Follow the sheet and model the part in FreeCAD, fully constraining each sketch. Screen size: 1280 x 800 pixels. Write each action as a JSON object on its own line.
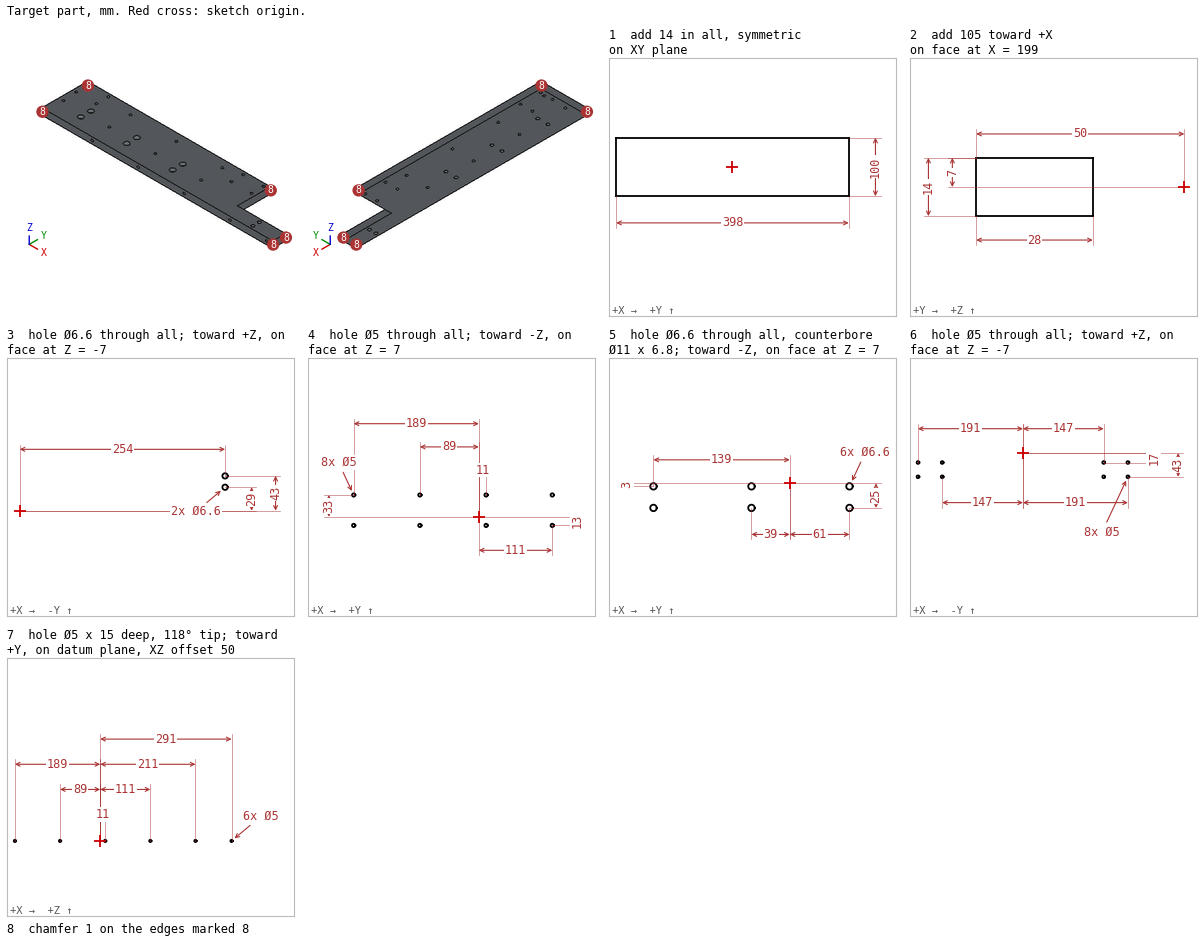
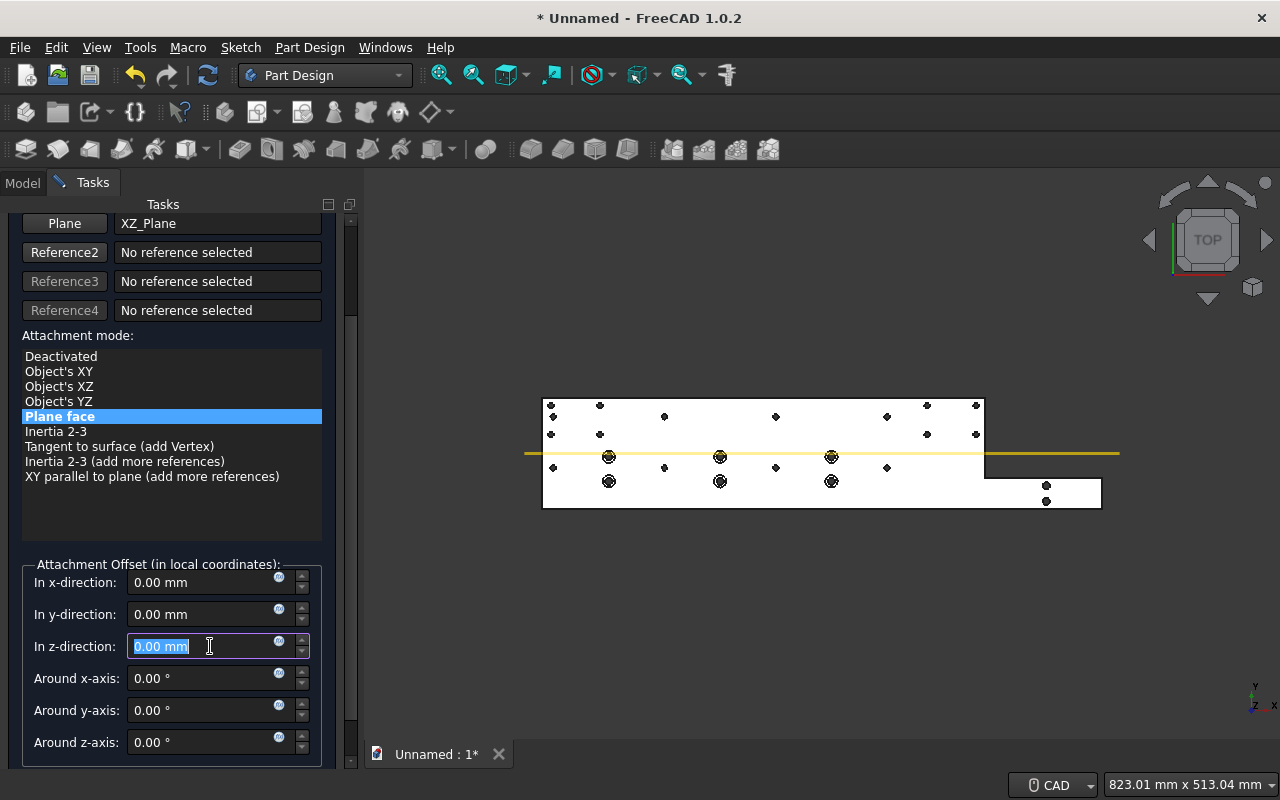
{"action": "type", "text": "50"}
{"action": "key", "text": "Tab"}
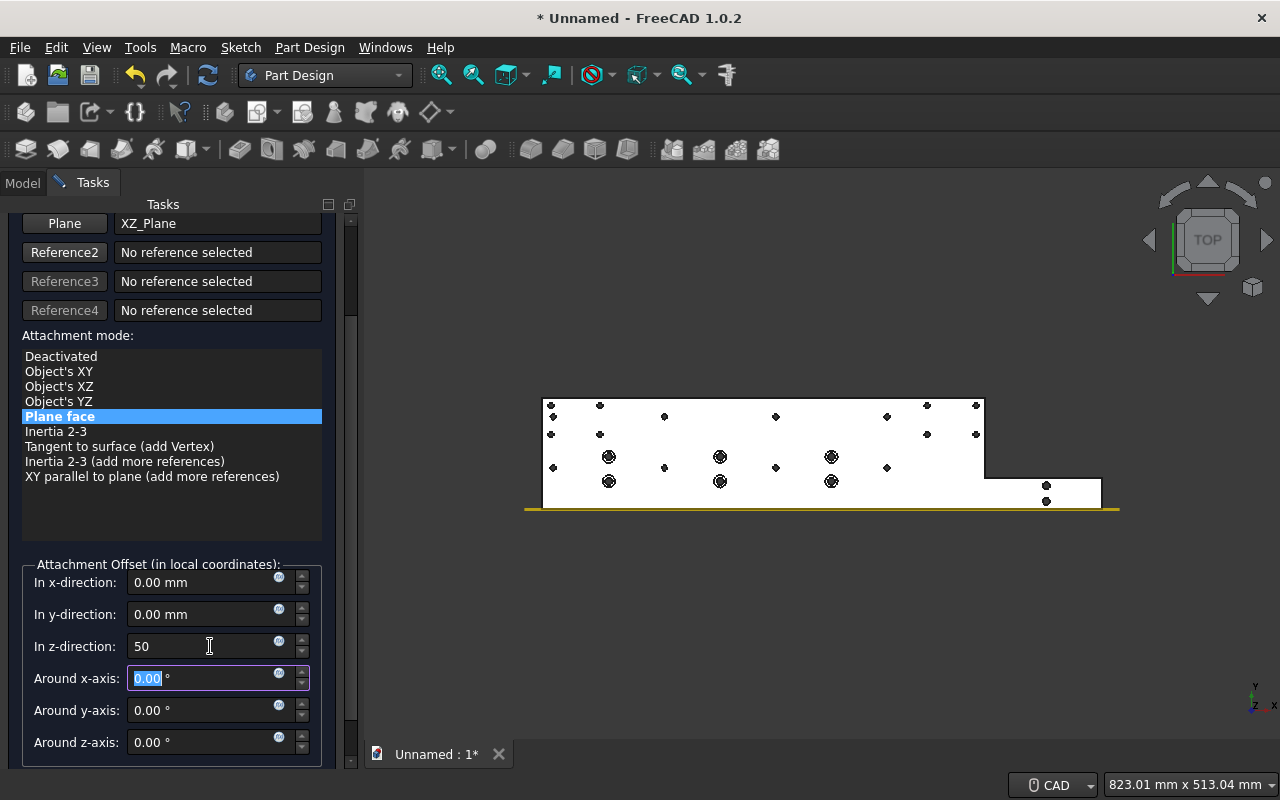
{"action": "scroll", "coordinate": [351, 491], "scroll_direction": "up", "scroll_amount": 3}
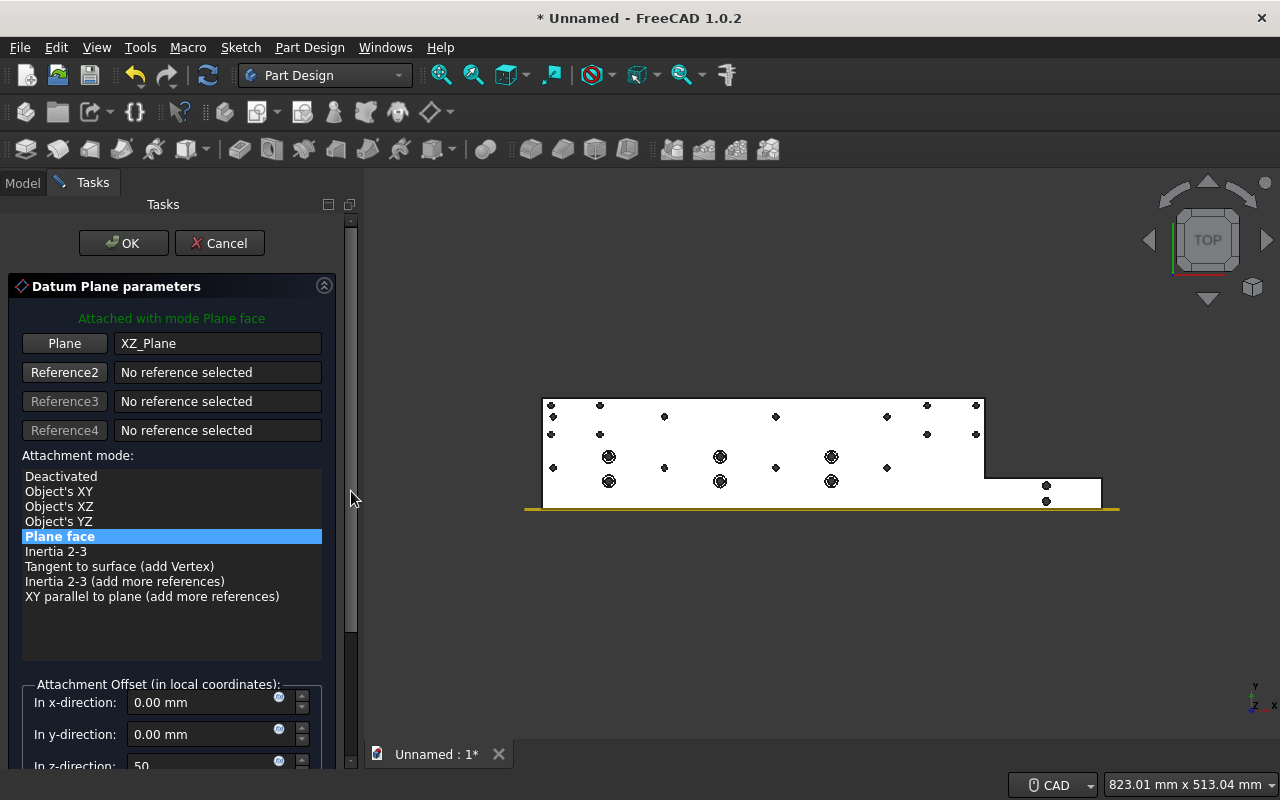
{"action": "left_click", "coordinate": [124, 243]}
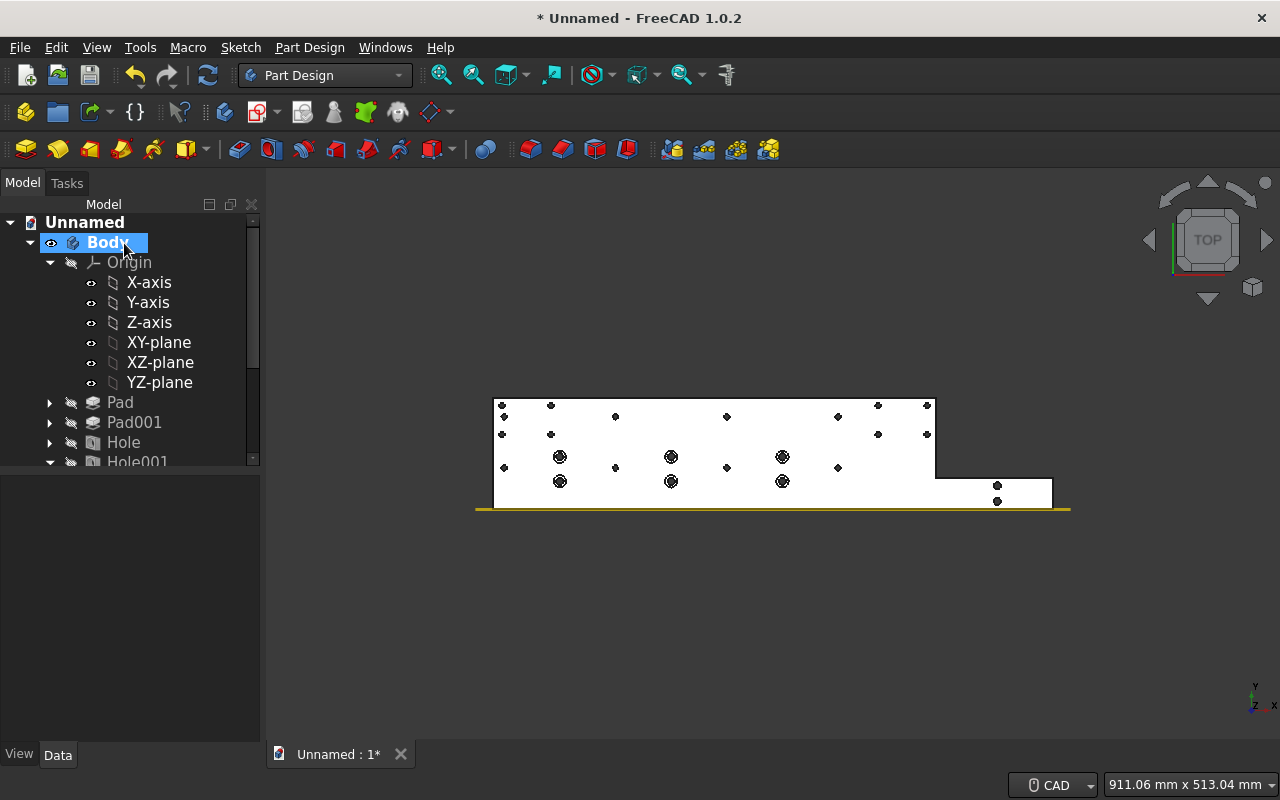
{"action": "scroll", "coordinate": [100, 338], "scroll_direction": "down", "scroll_amount": 3}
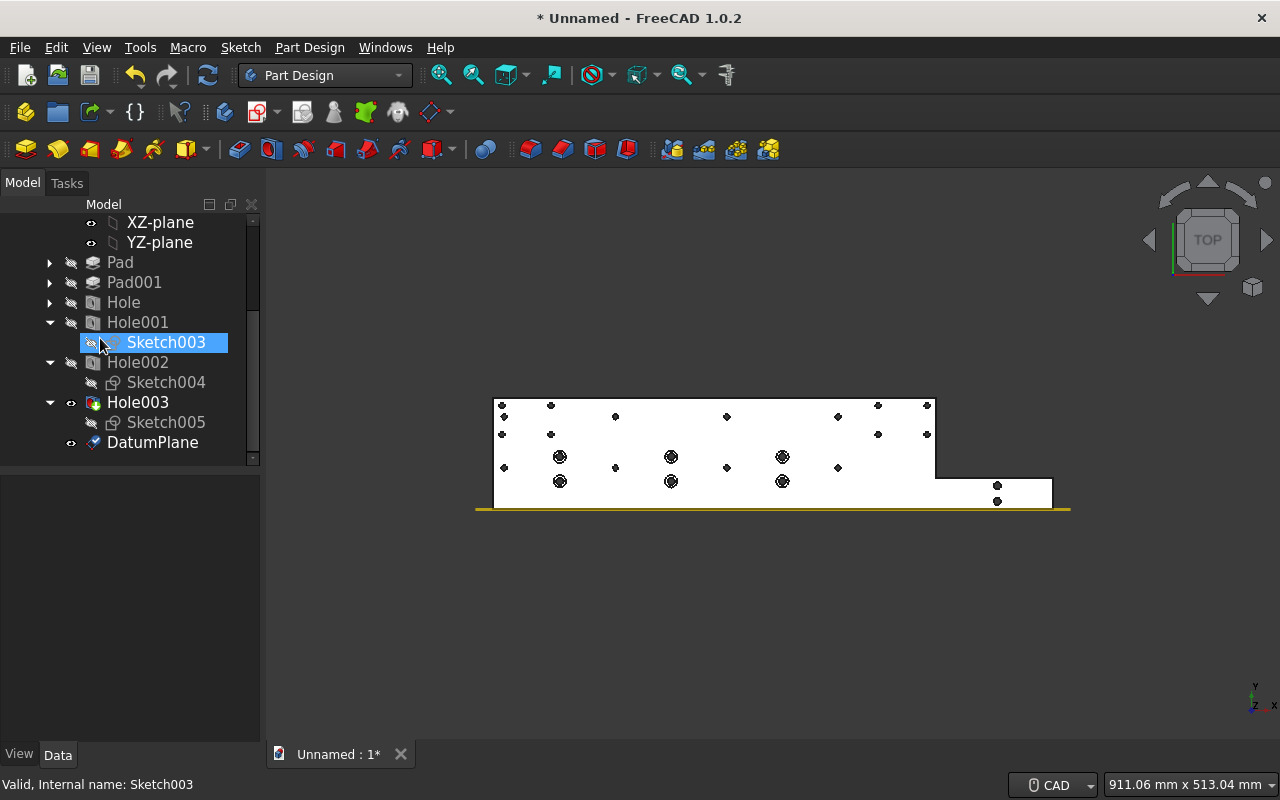
{"action": "left_click", "coordinate": [116, 443]}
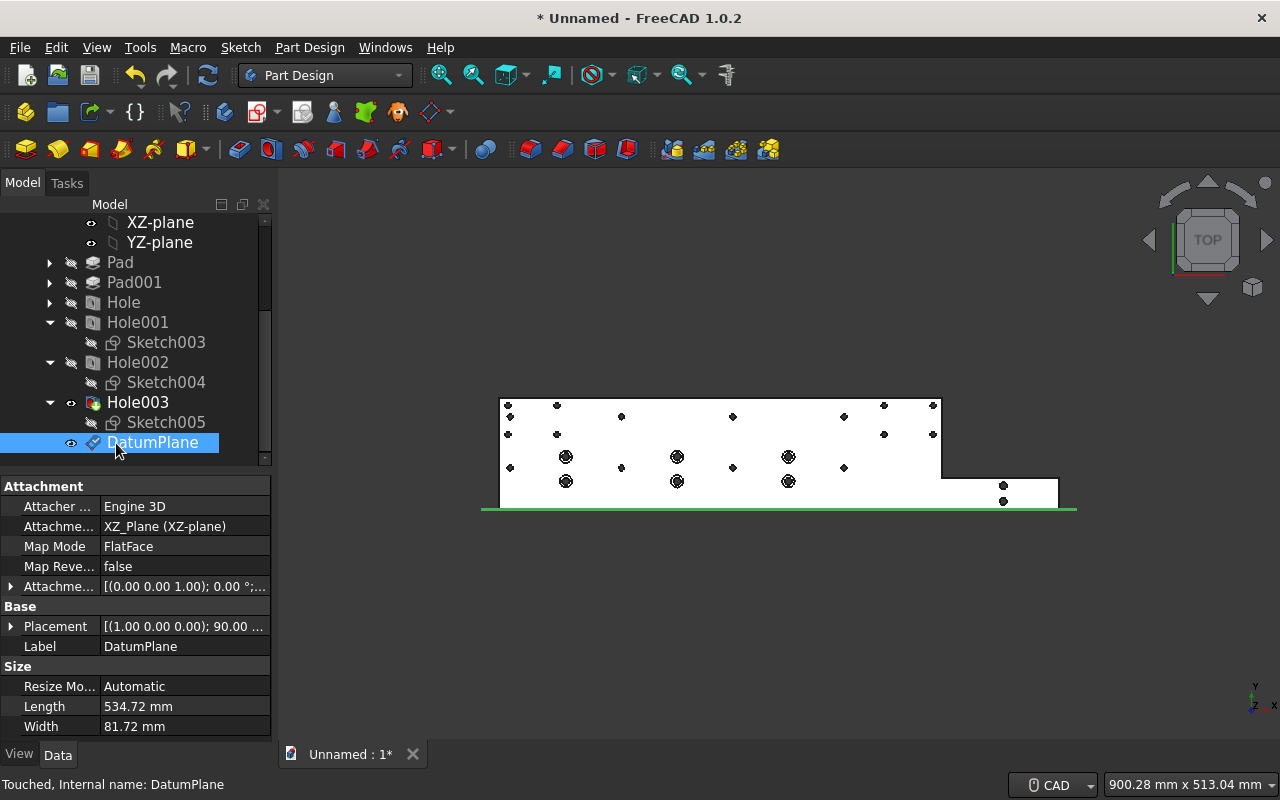
{"action": "left_click", "coordinate": [258, 112]}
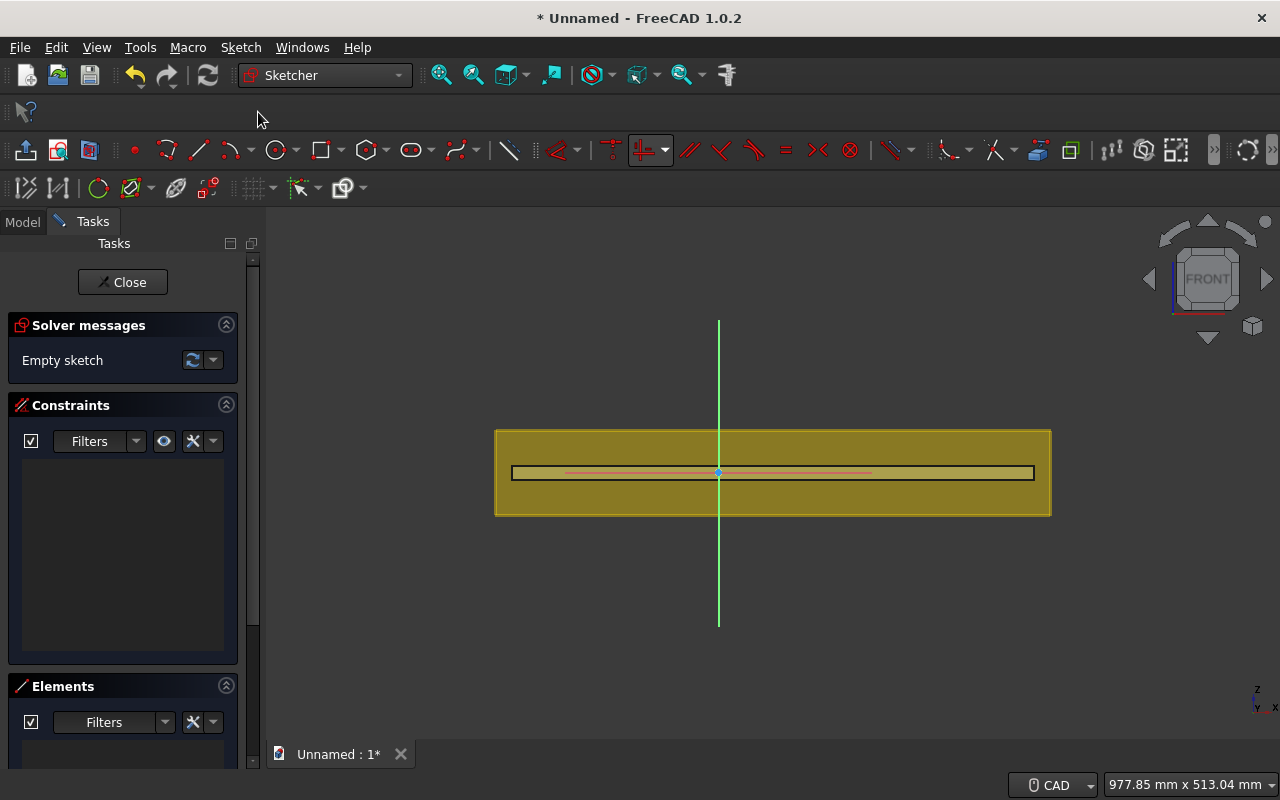
{"action": "left_click", "coordinate": [276, 150]}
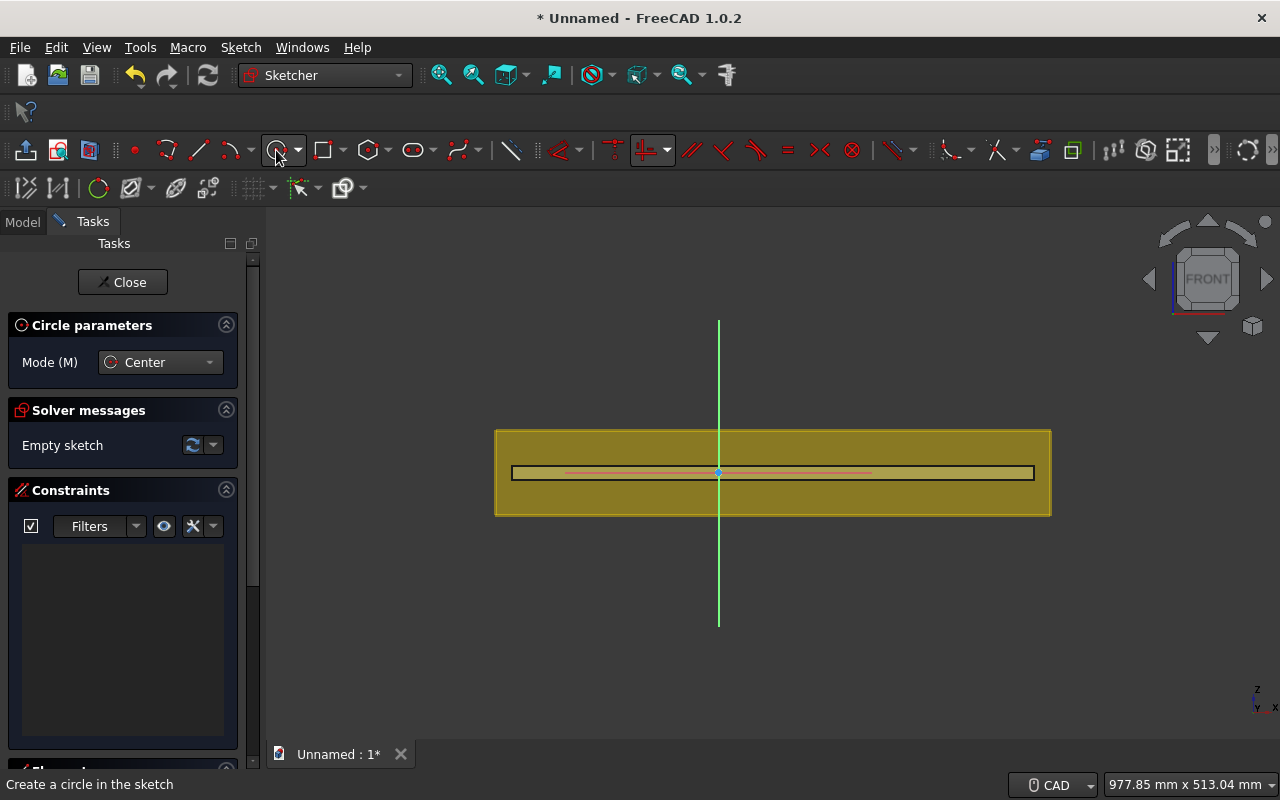
{"action": "scroll", "coordinate": [1020, 473], "scroll_direction": "up", "scroll_amount": 11}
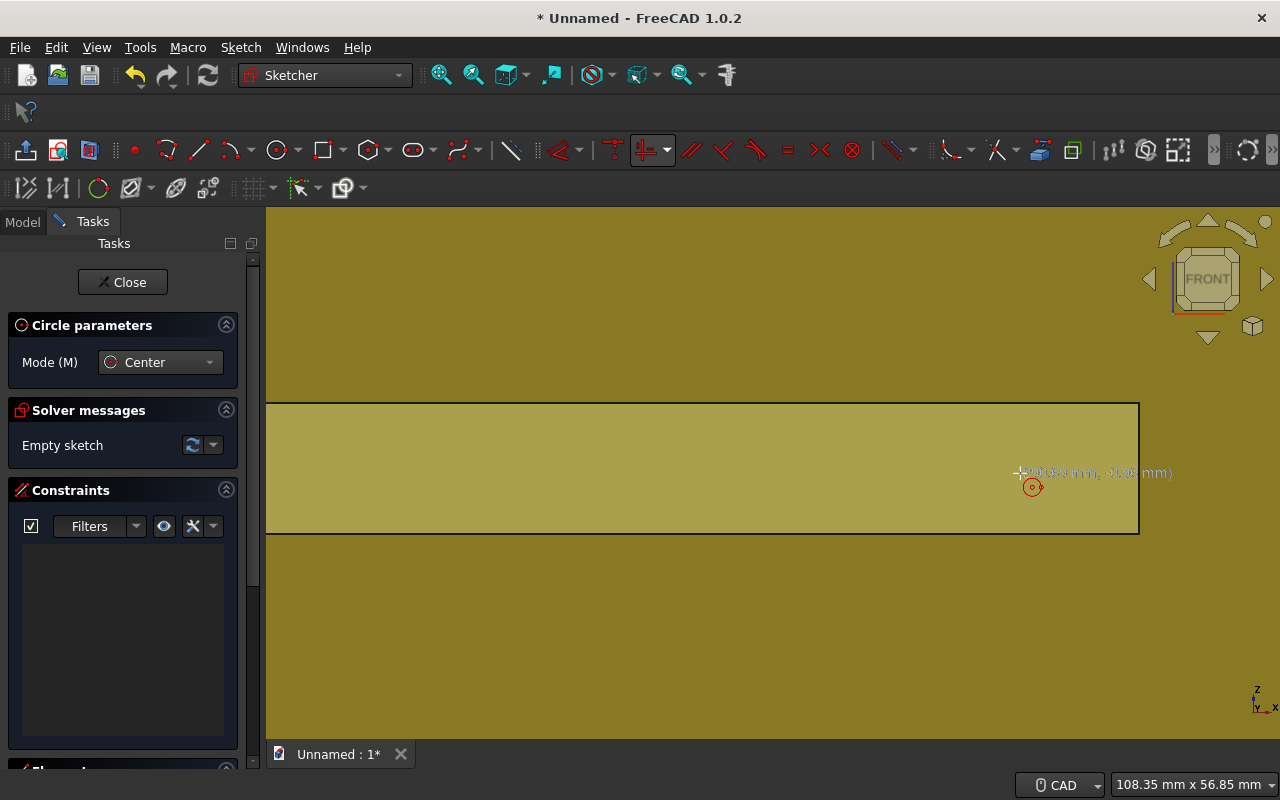
{"action": "scroll", "coordinate": [1007, 474], "scroll_direction": "down", "scroll_amount": 10}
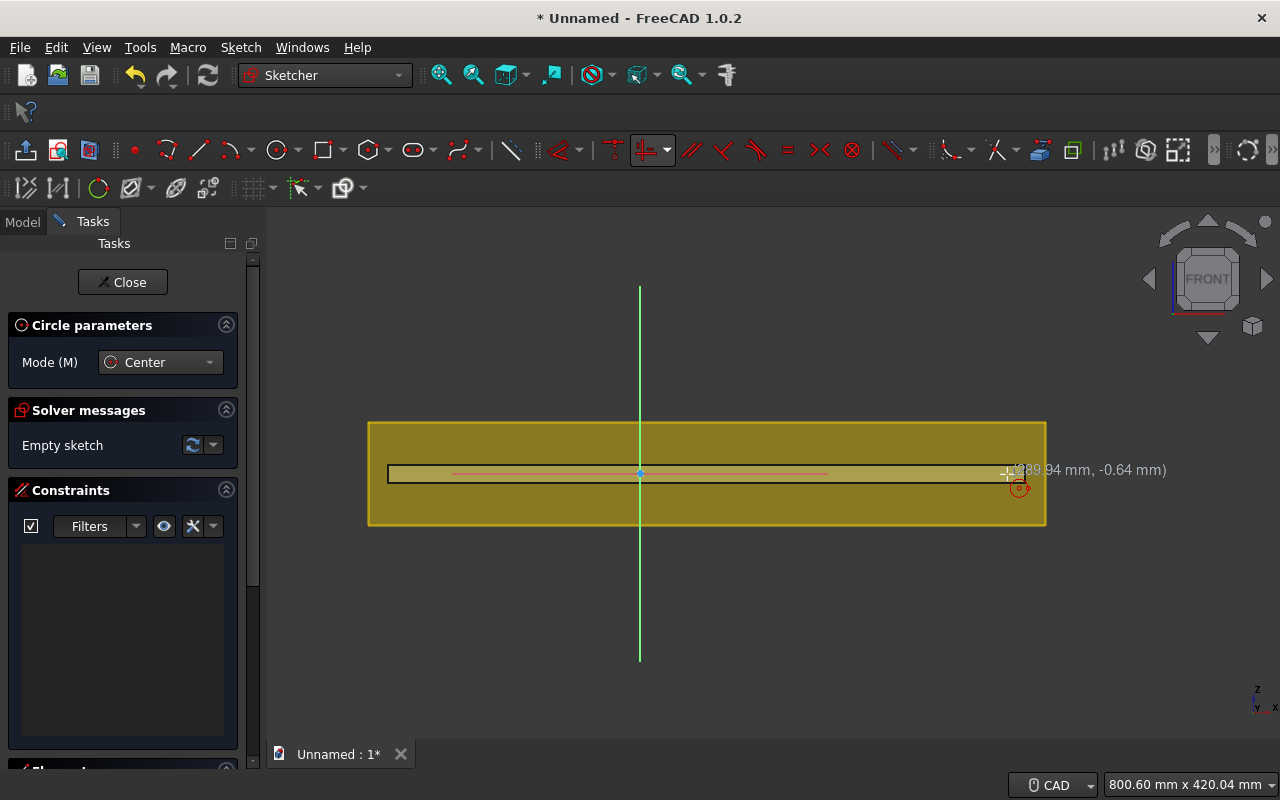
{"action": "left_click", "coordinate": [1009, 474]}